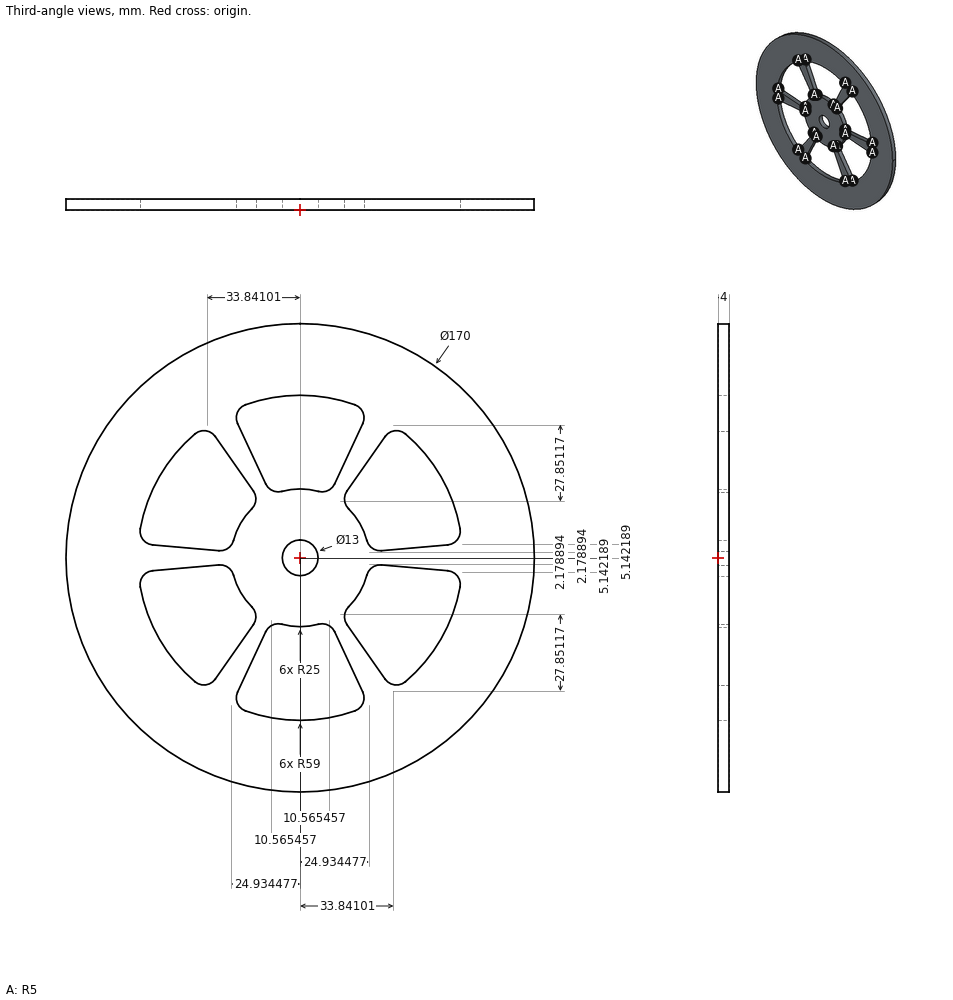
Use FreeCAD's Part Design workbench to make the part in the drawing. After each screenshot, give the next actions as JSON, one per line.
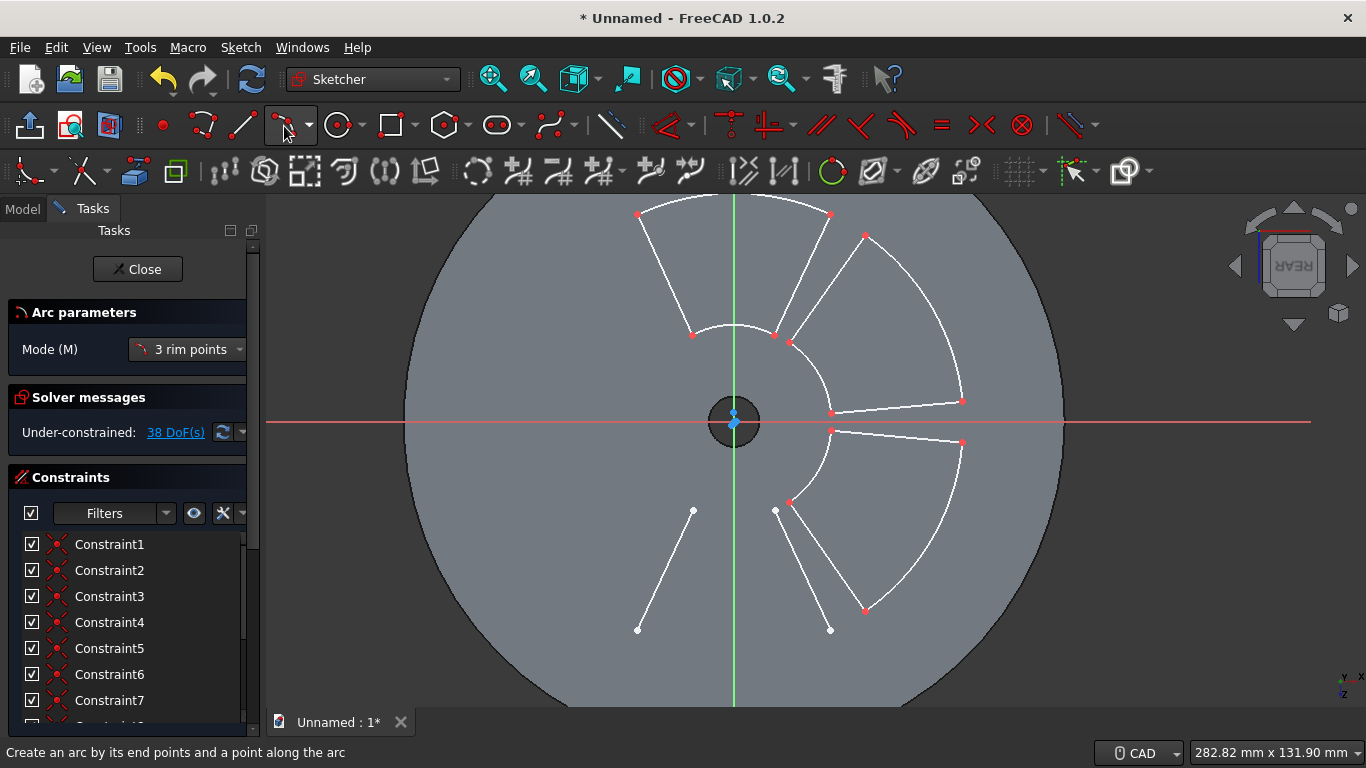
{"action": "left_click", "coordinate": [775, 511]}
{"action": "left_click", "coordinate": [693, 511]}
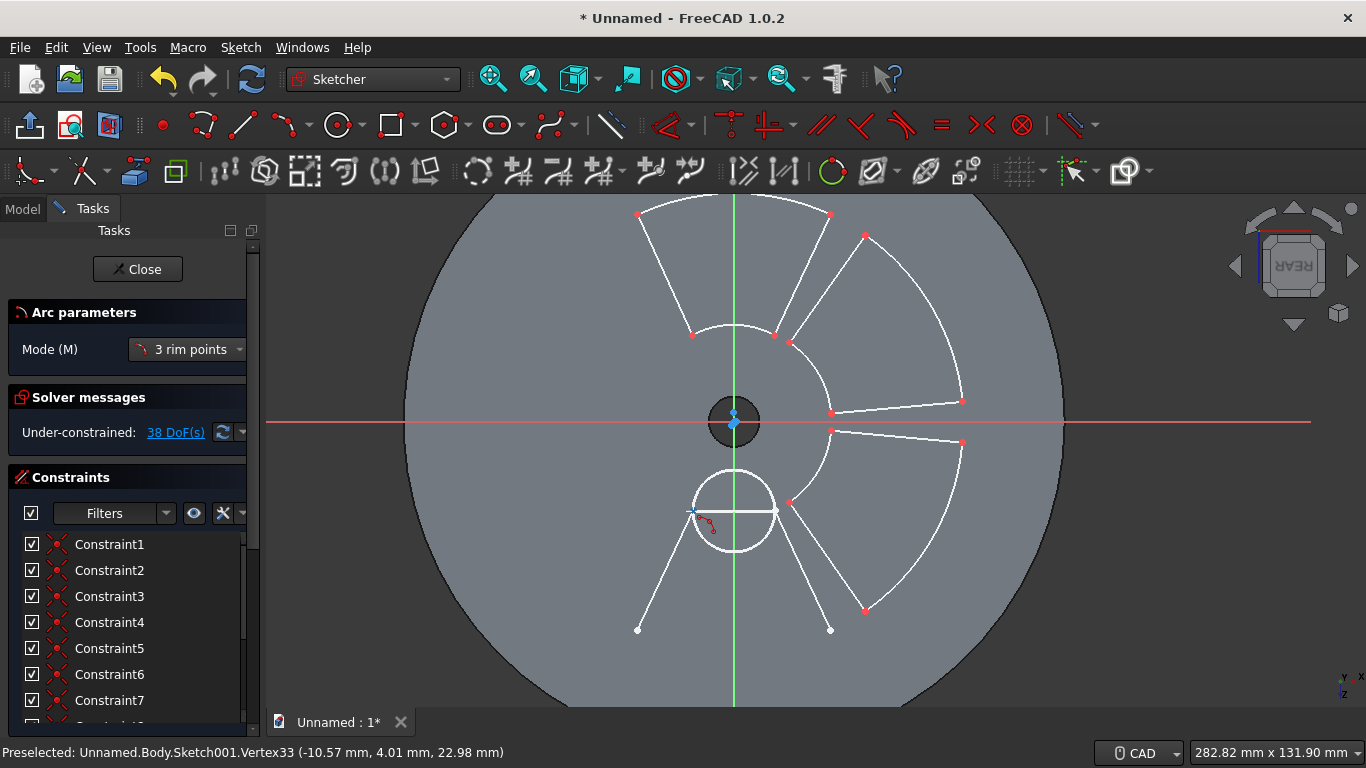
{"action": "scroll", "coordinate": [726, 518], "scroll_direction": "up", "scroll_amount": 4}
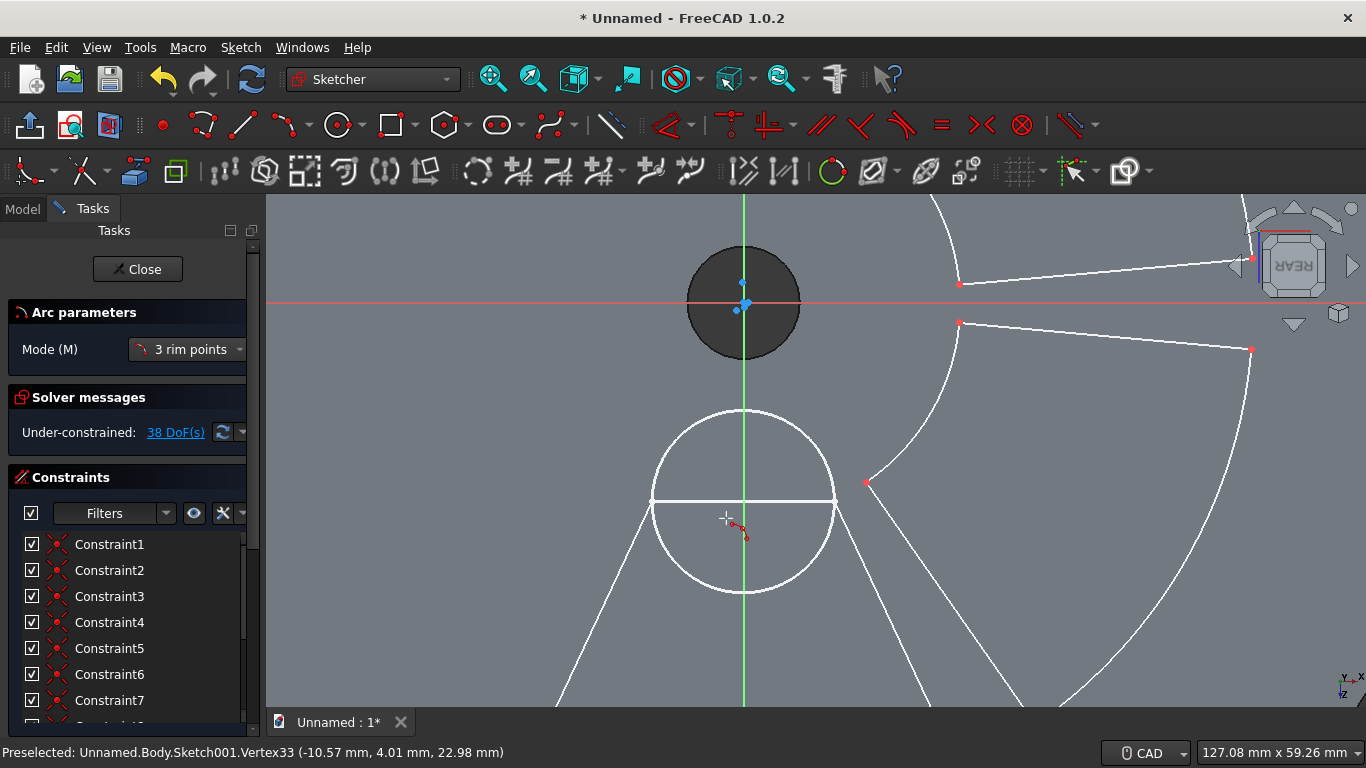
{"action": "left_click", "coordinate": [725, 518]}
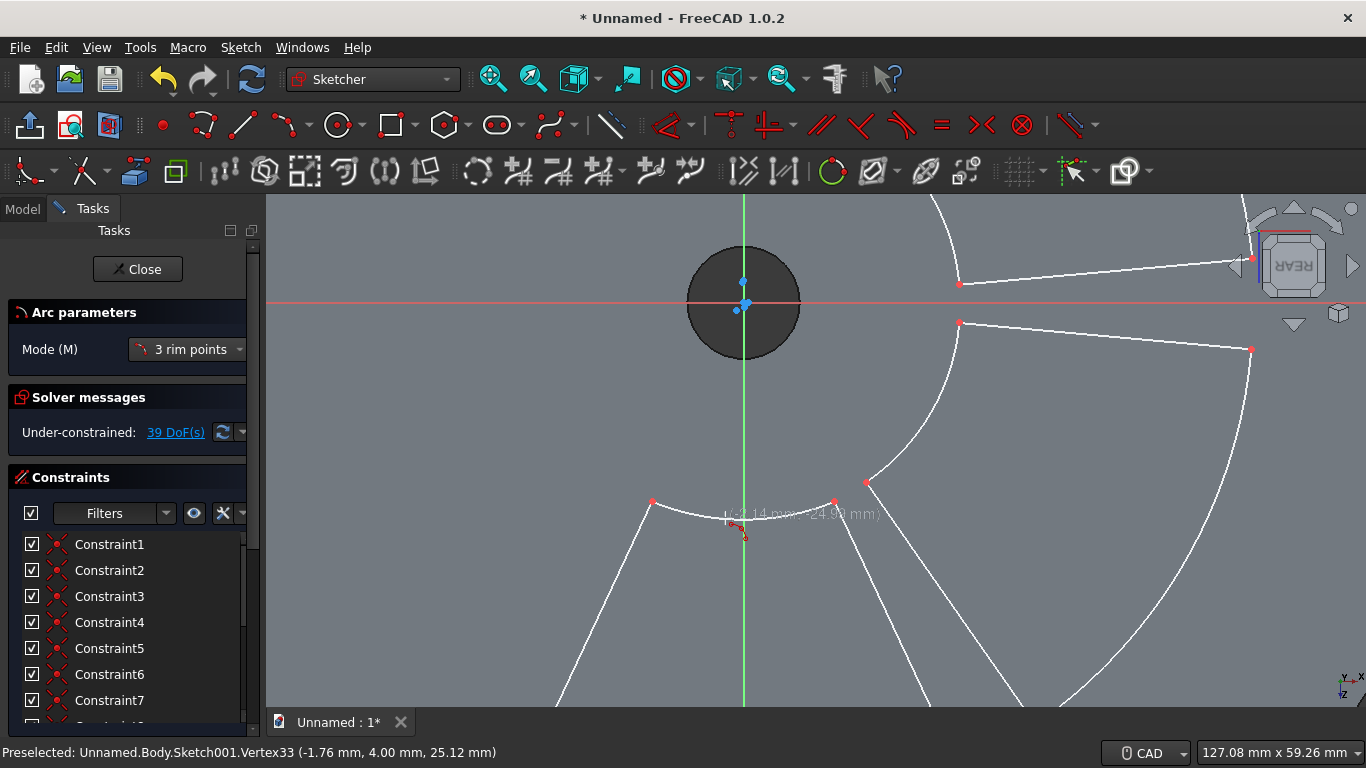
{"action": "scroll", "coordinate": [749, 514], "scroll_direction": "down", "scroll_amount": 6}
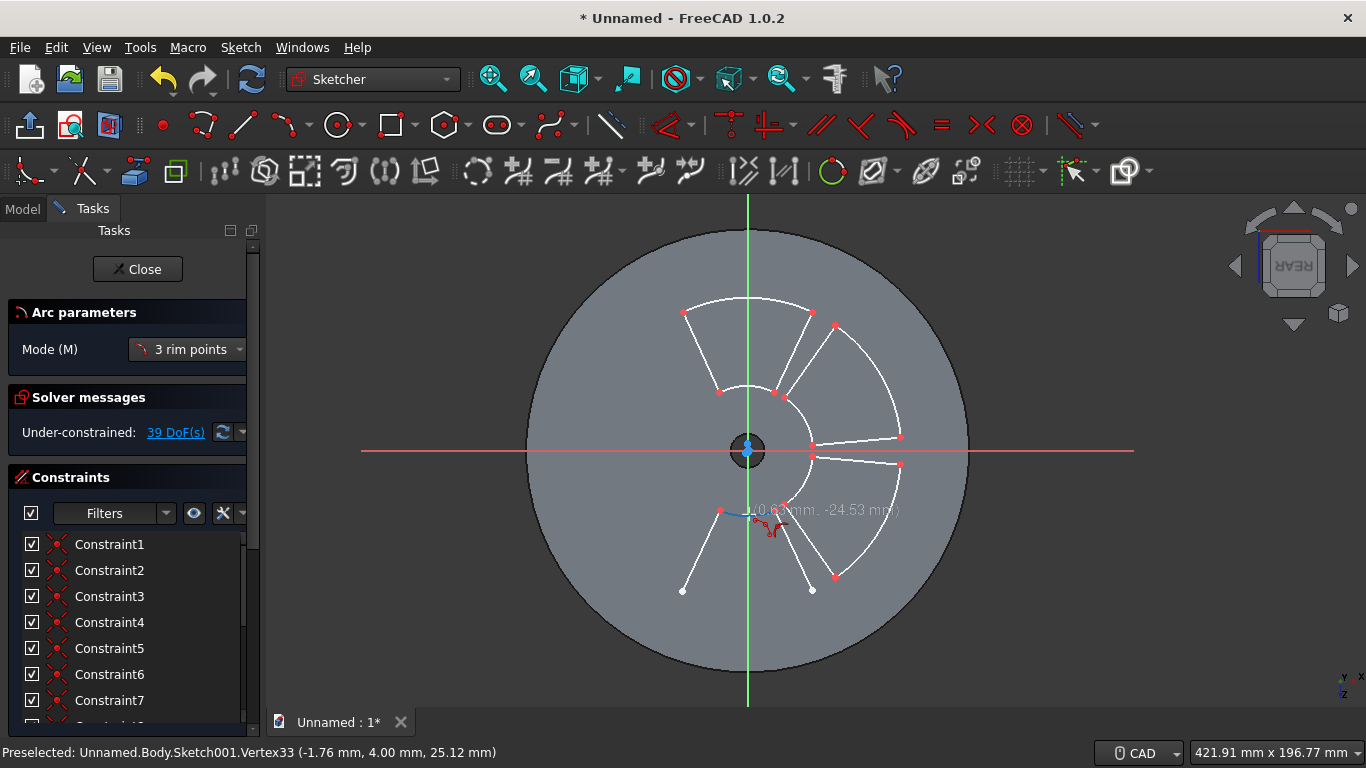
{"action": "left_click", "coordinate": [683, 591]}
{"action": "left_click", "coordinate": [813, 591]}
{"action": "left_click", "coordinate": [761, 604]}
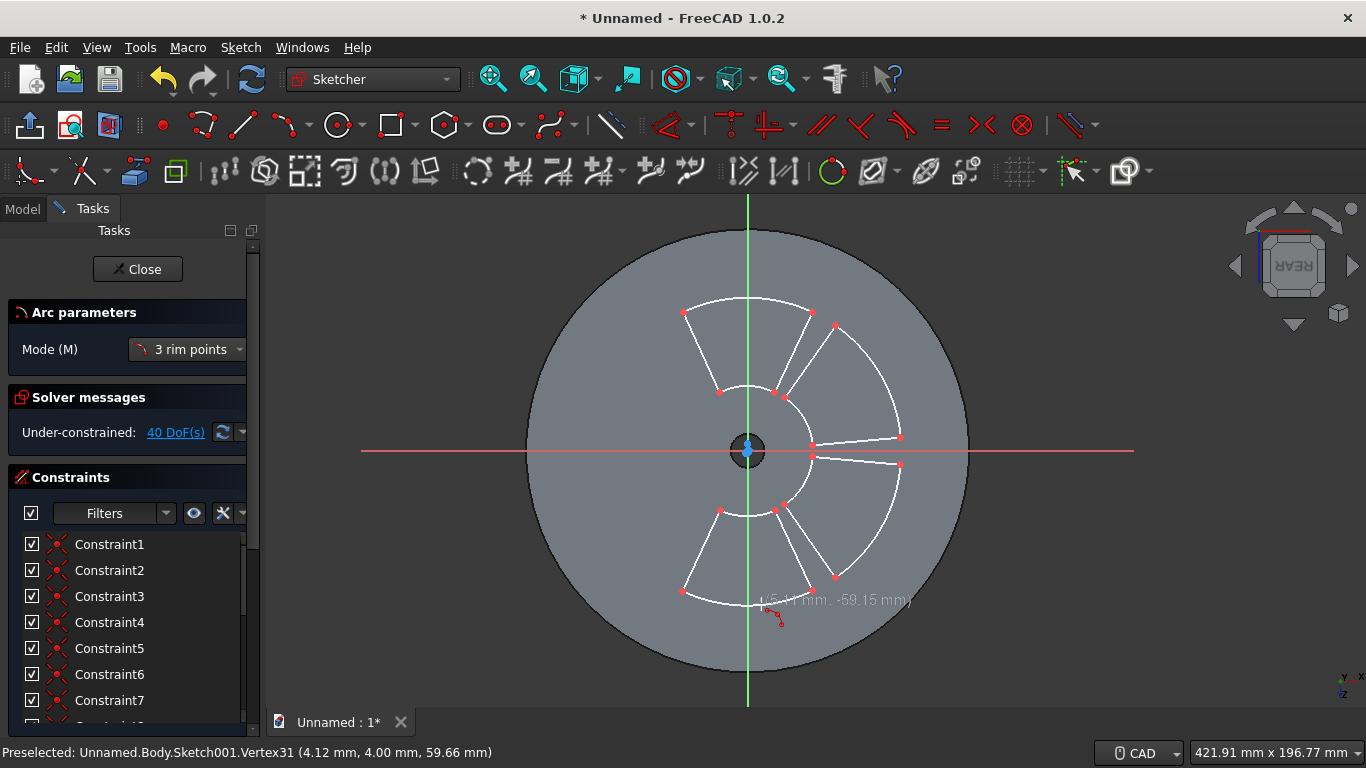
{"action": "left_click", "coordinate": [244, 126]}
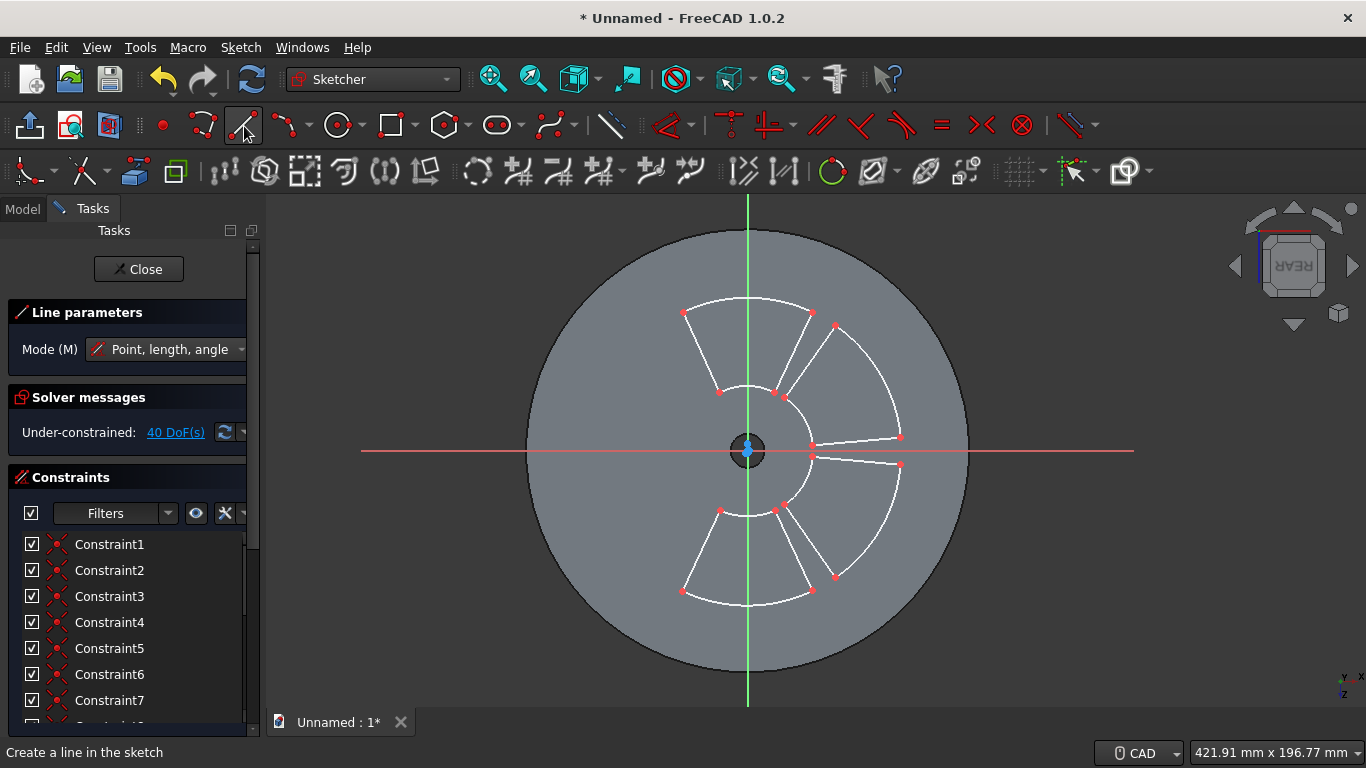
{"action": "left_click", "coordinate": [659, 577]}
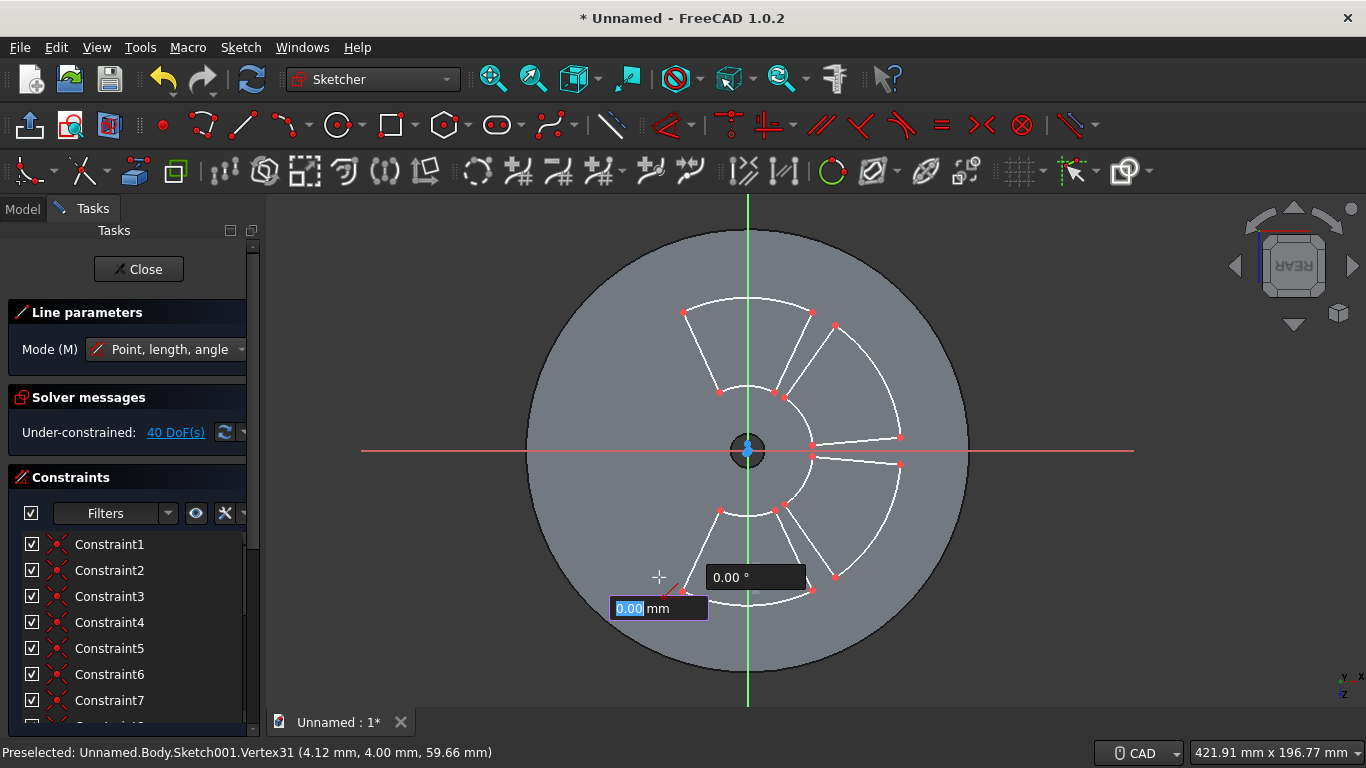
{"action": "scroll", "coordinate": [710, 504], "scroll_direction": "up", "scroll_amount": 2}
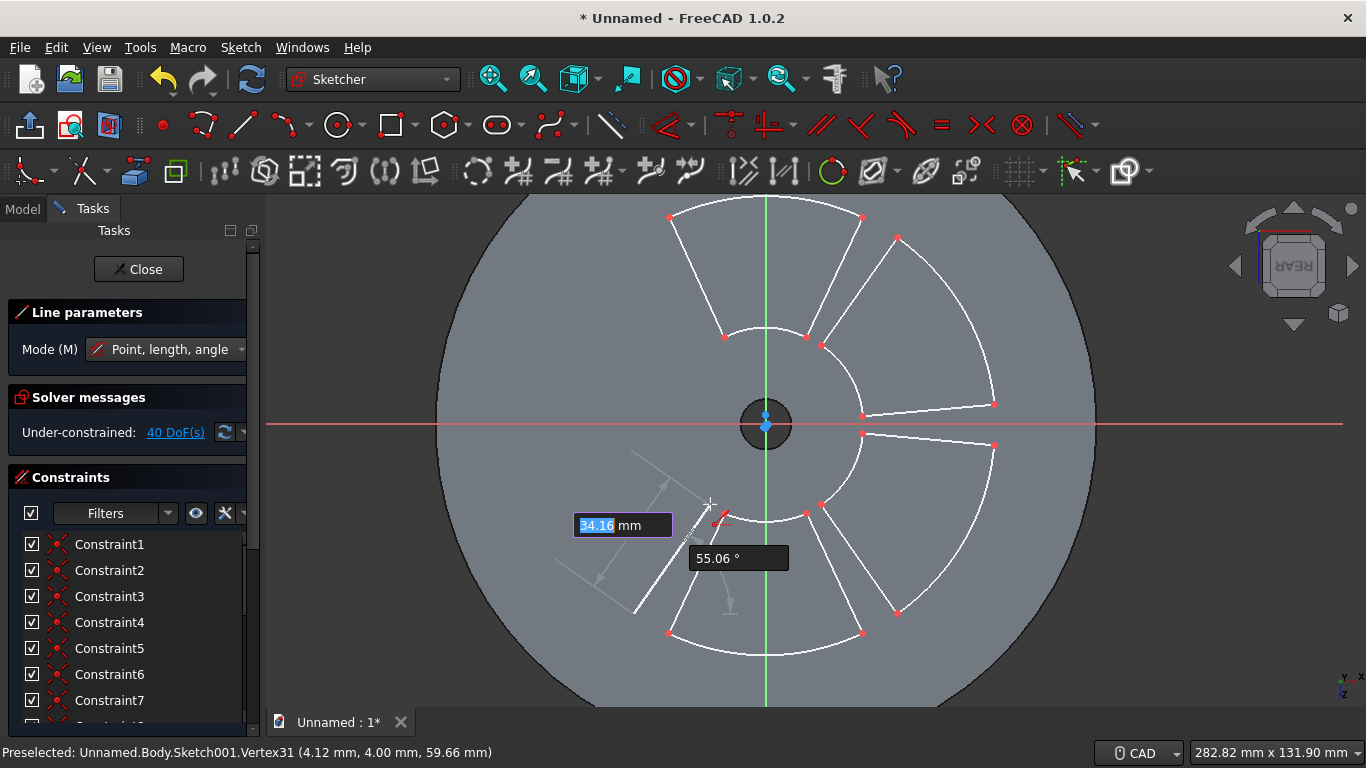
{"action": "left_click", "coordinate": [710, 504]}